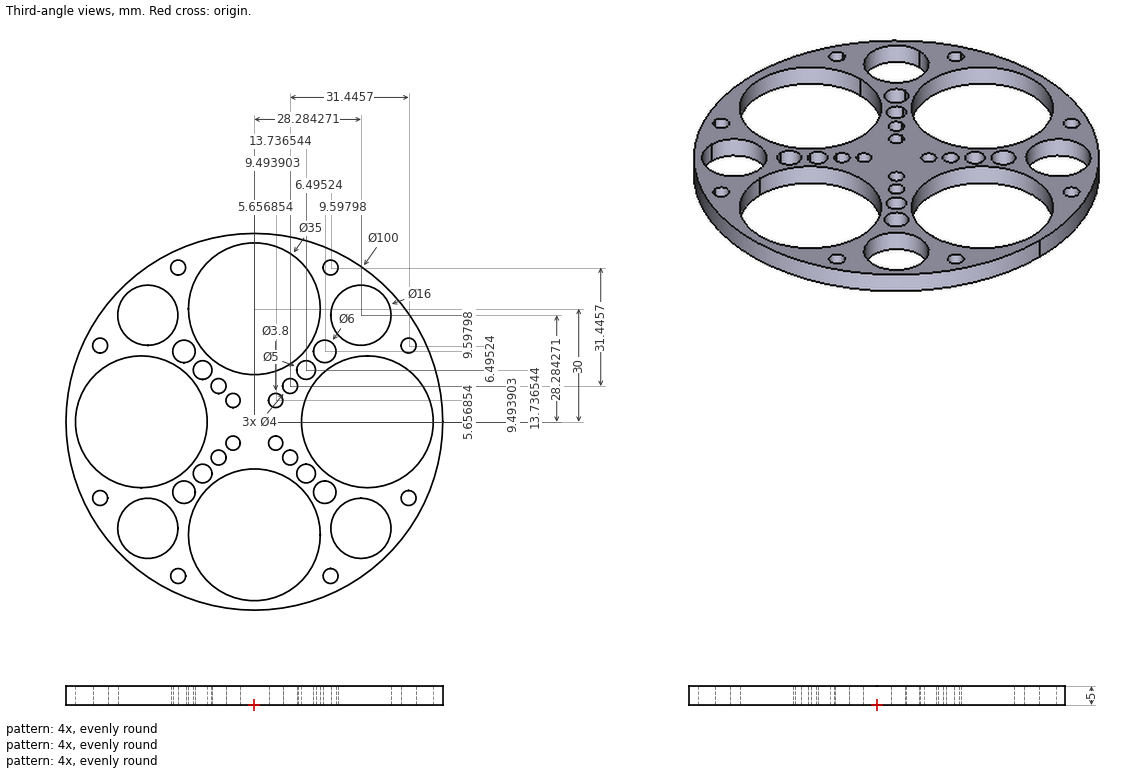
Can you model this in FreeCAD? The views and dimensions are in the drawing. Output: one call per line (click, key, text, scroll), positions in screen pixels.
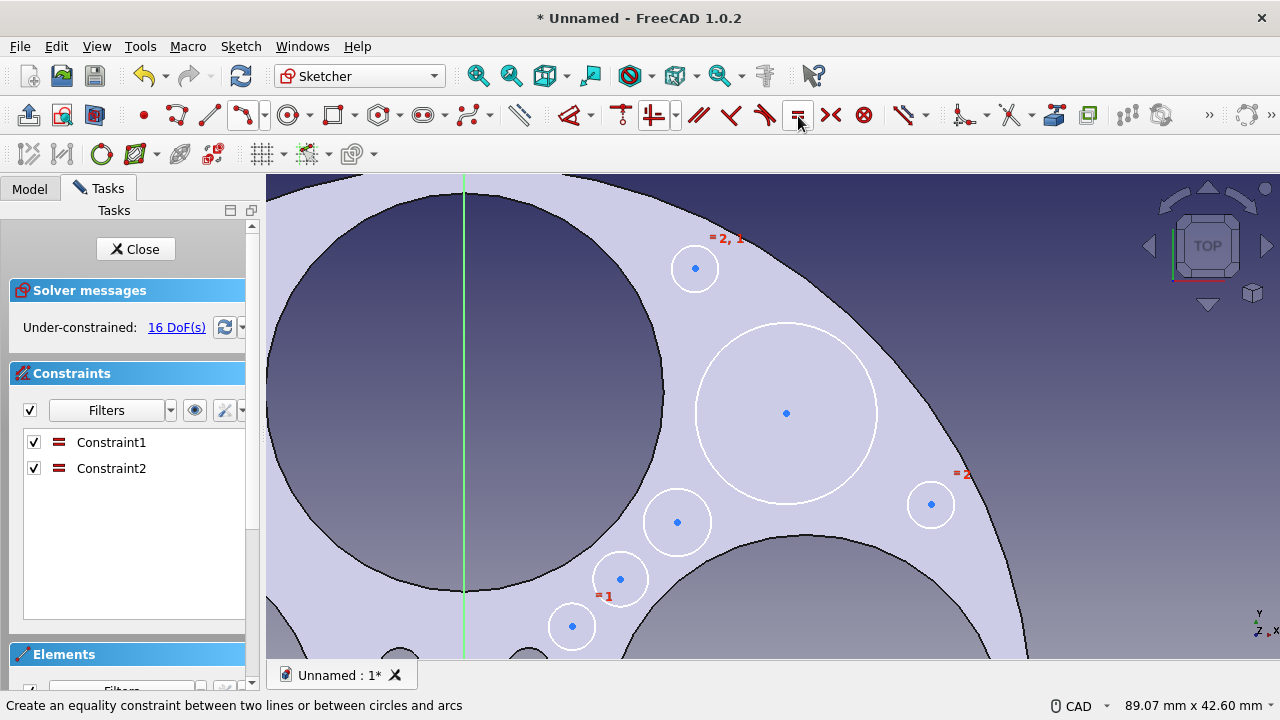
click(568, 116)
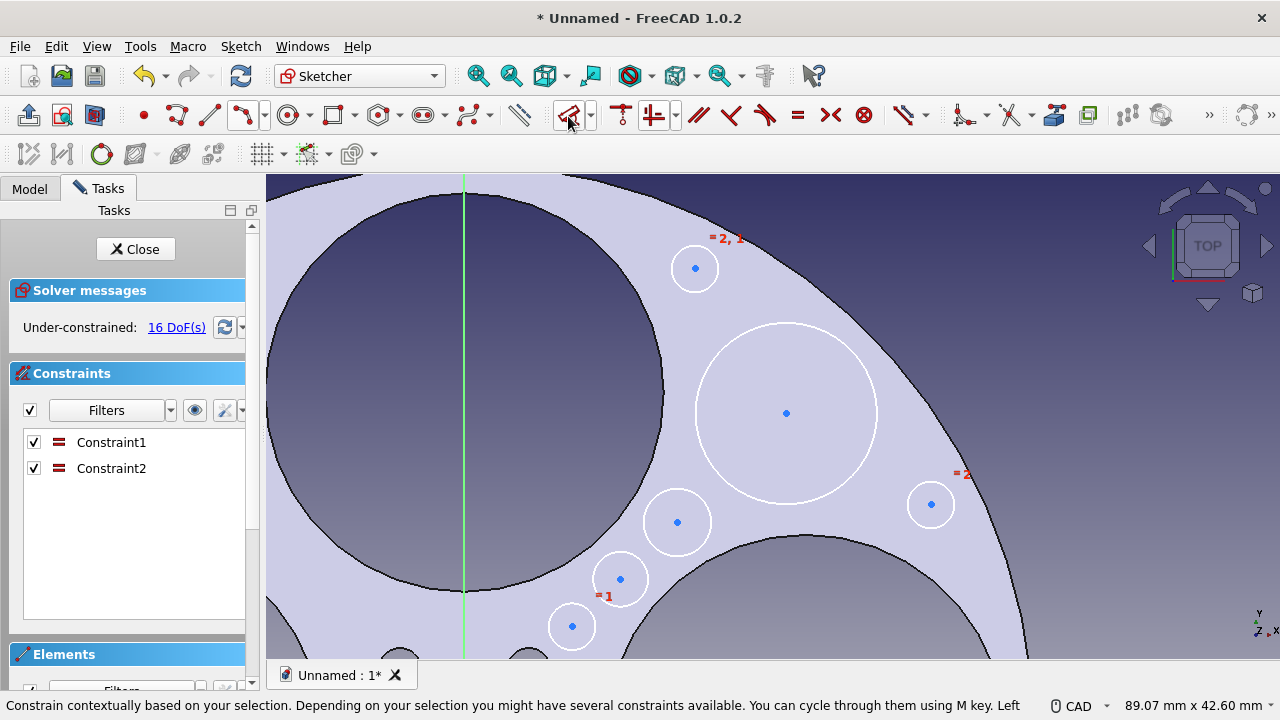
click(850, 349)
click(872, 326)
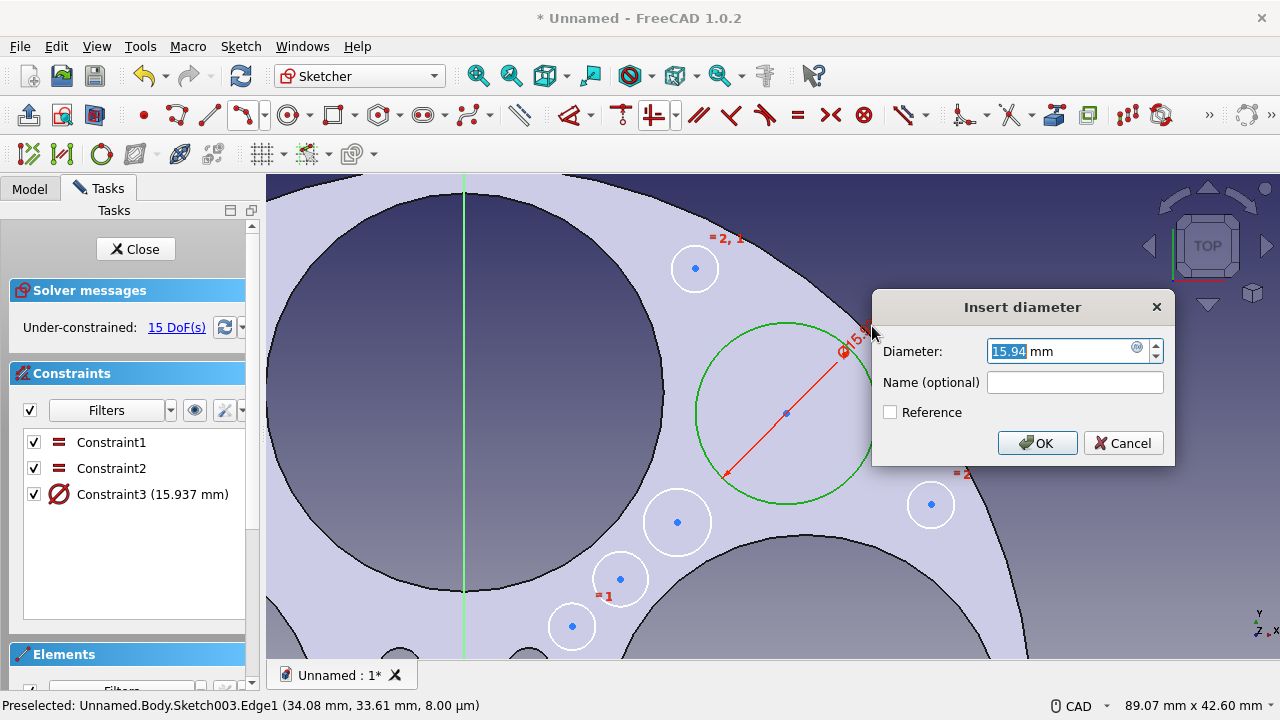
text(16)
key(Return)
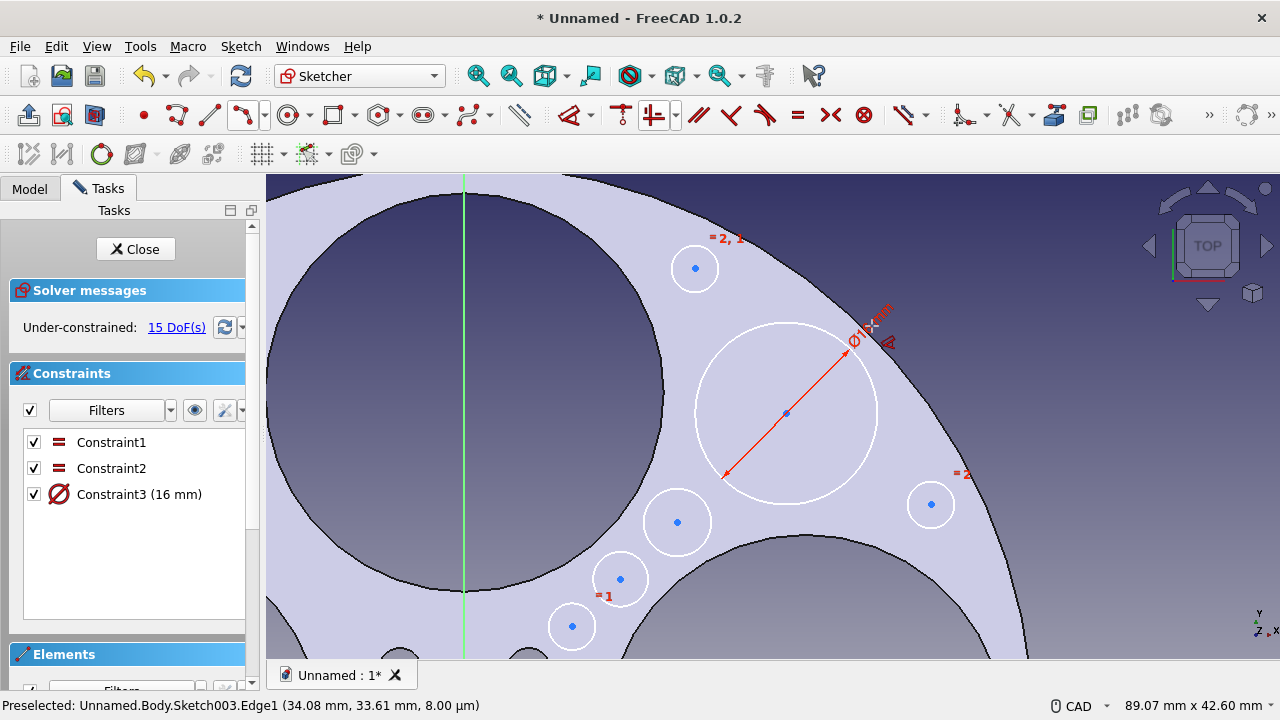
click(701, 499)
click(741, 537)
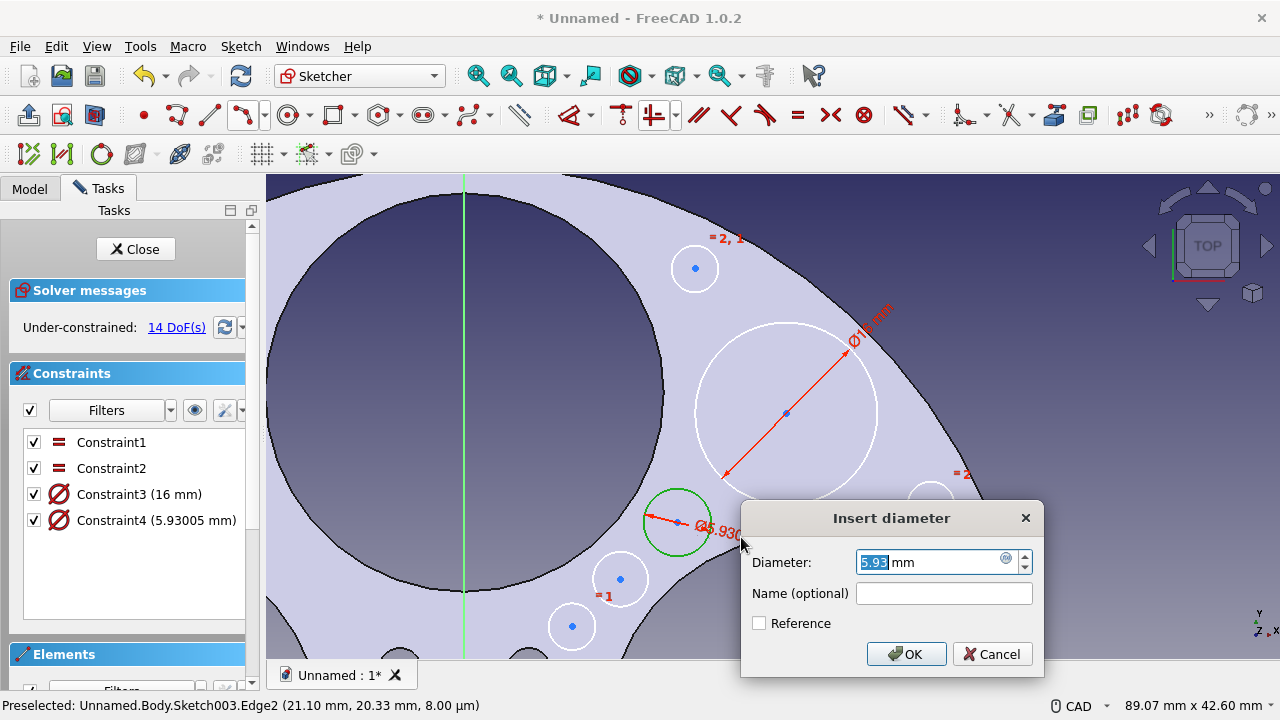
text(6)
key(Return)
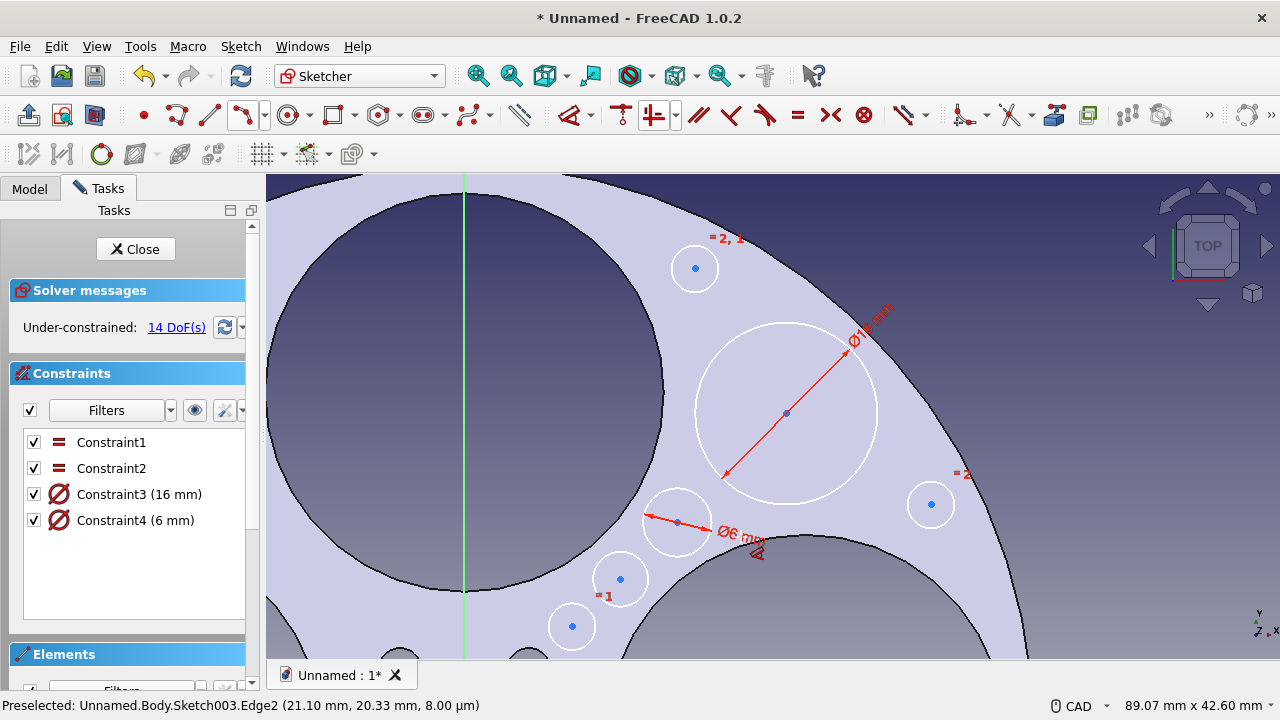
click(640, 560)
click(663, 537)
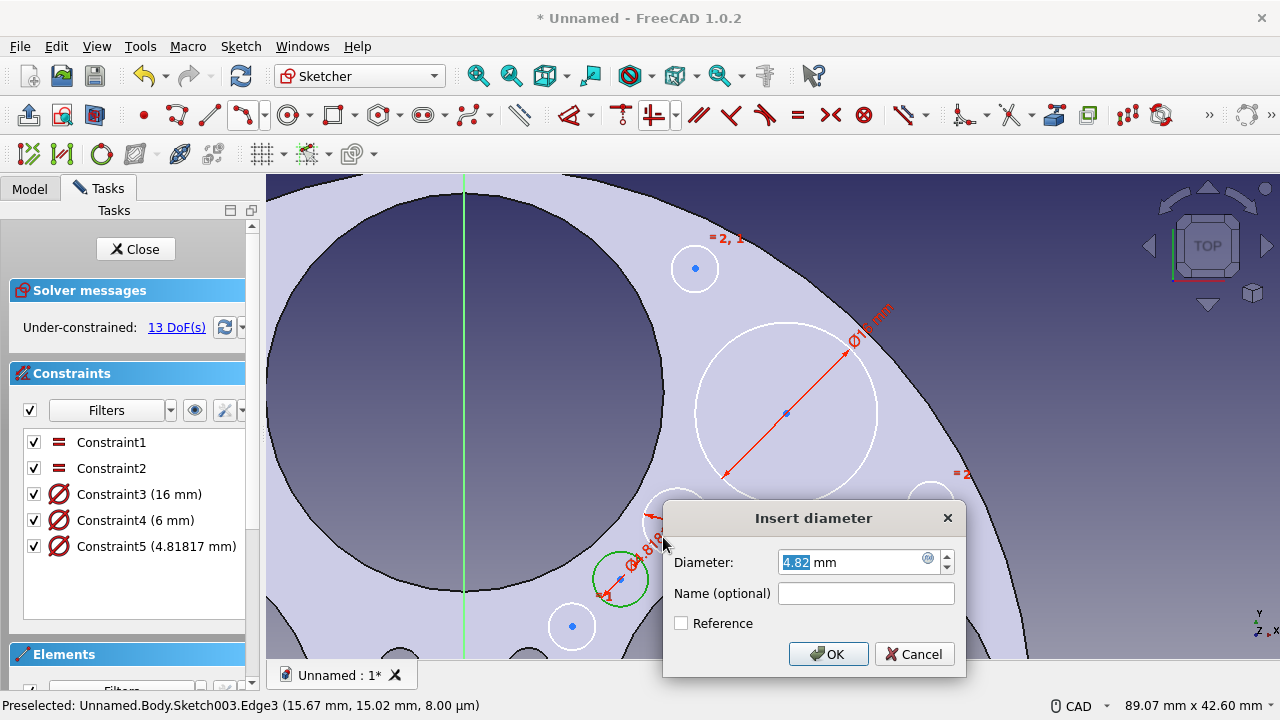
text(5)
key(Return)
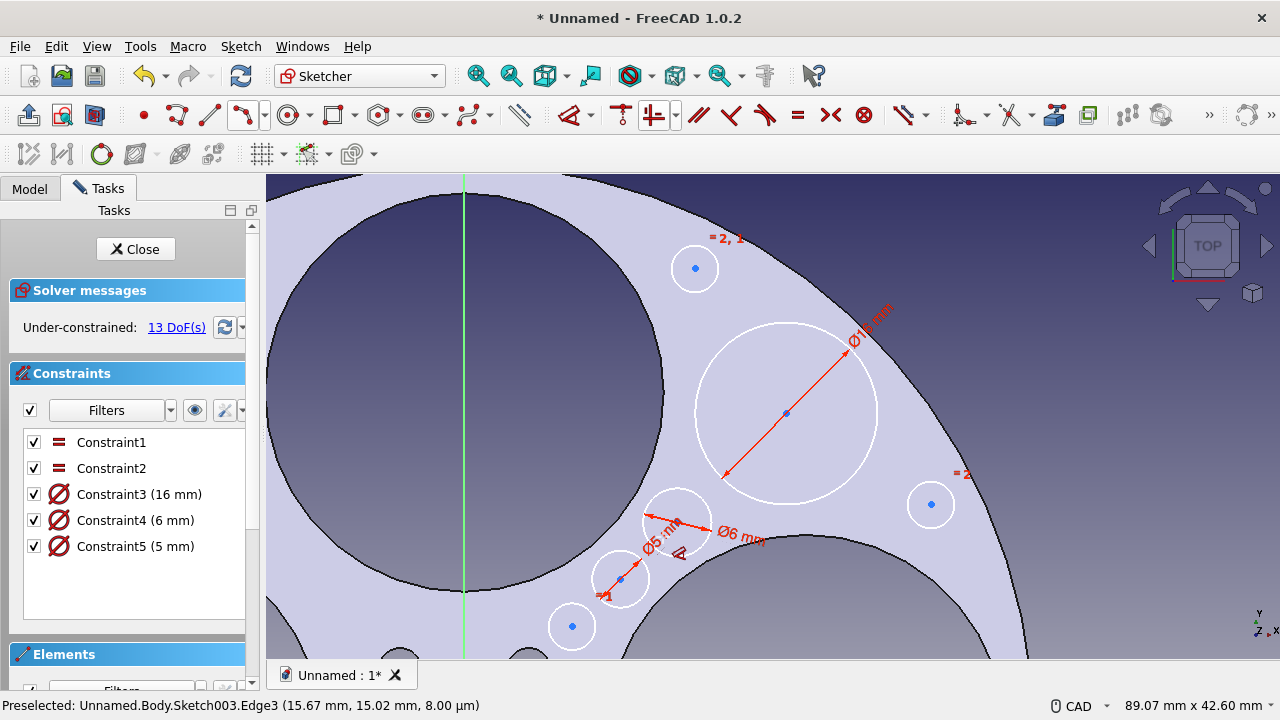
click(589, 610)
click(612, 587)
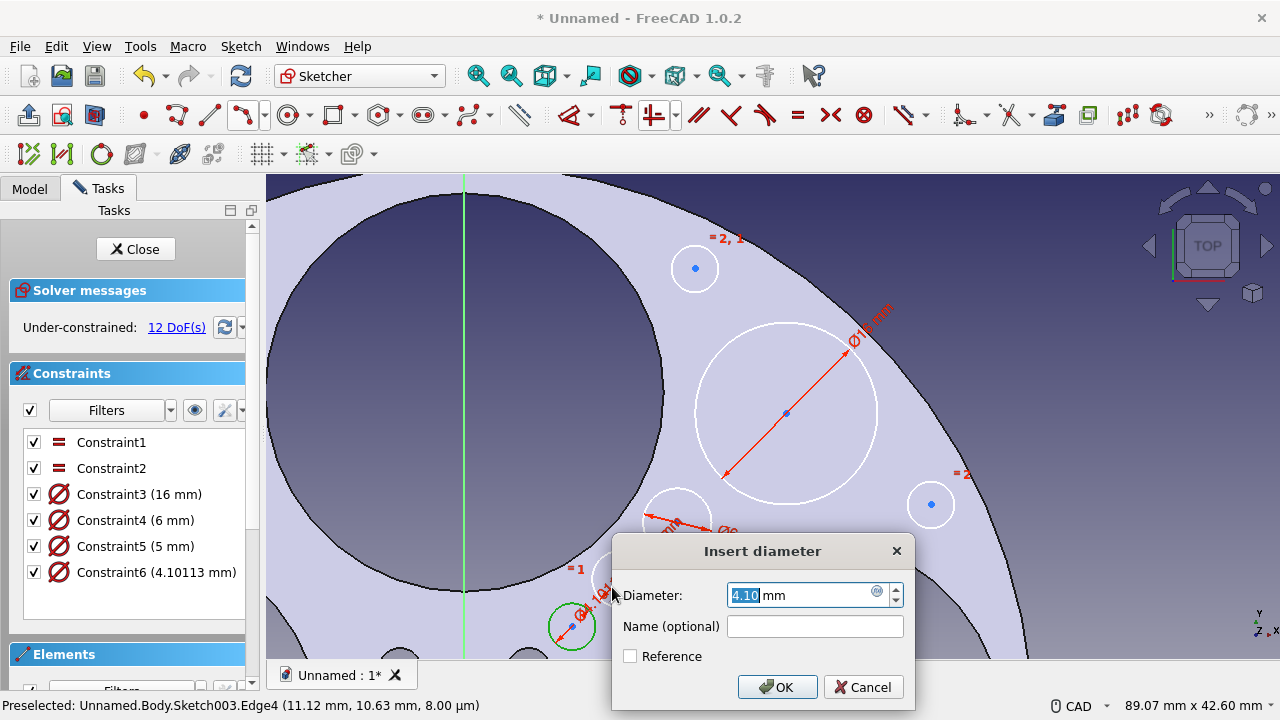
text(4)
key(Return)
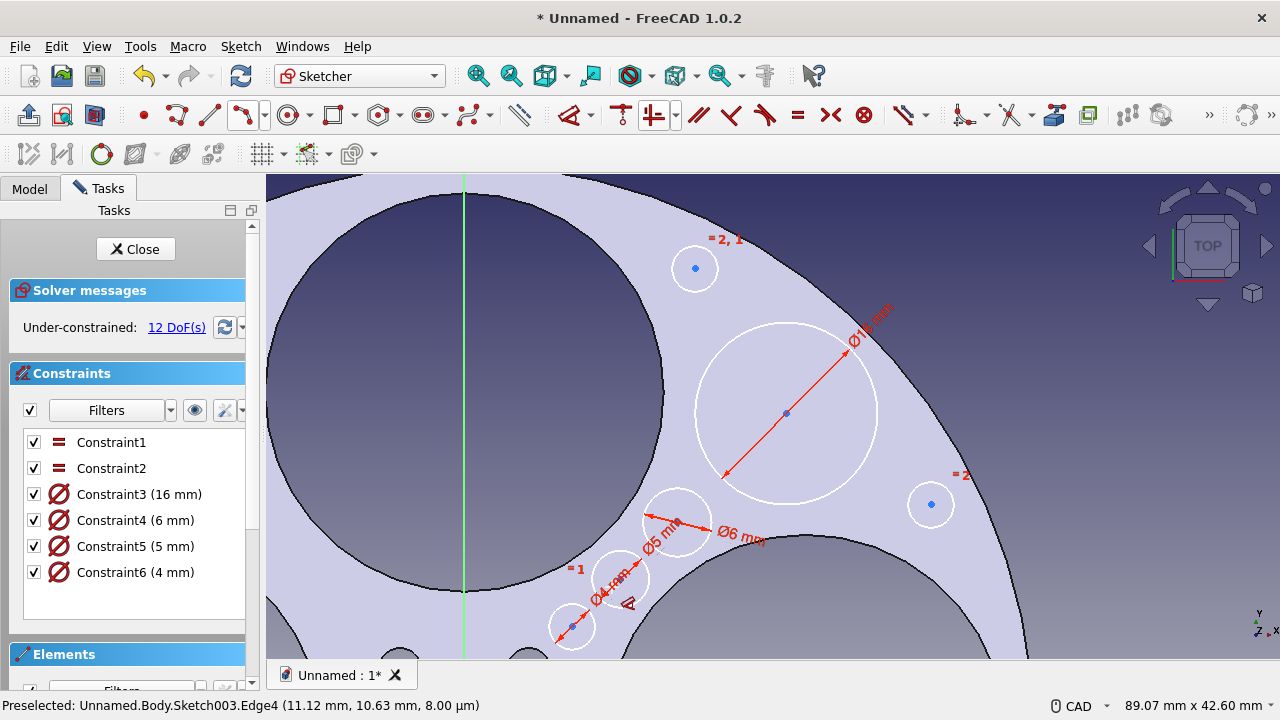
click(572, 627)
click(518, 593)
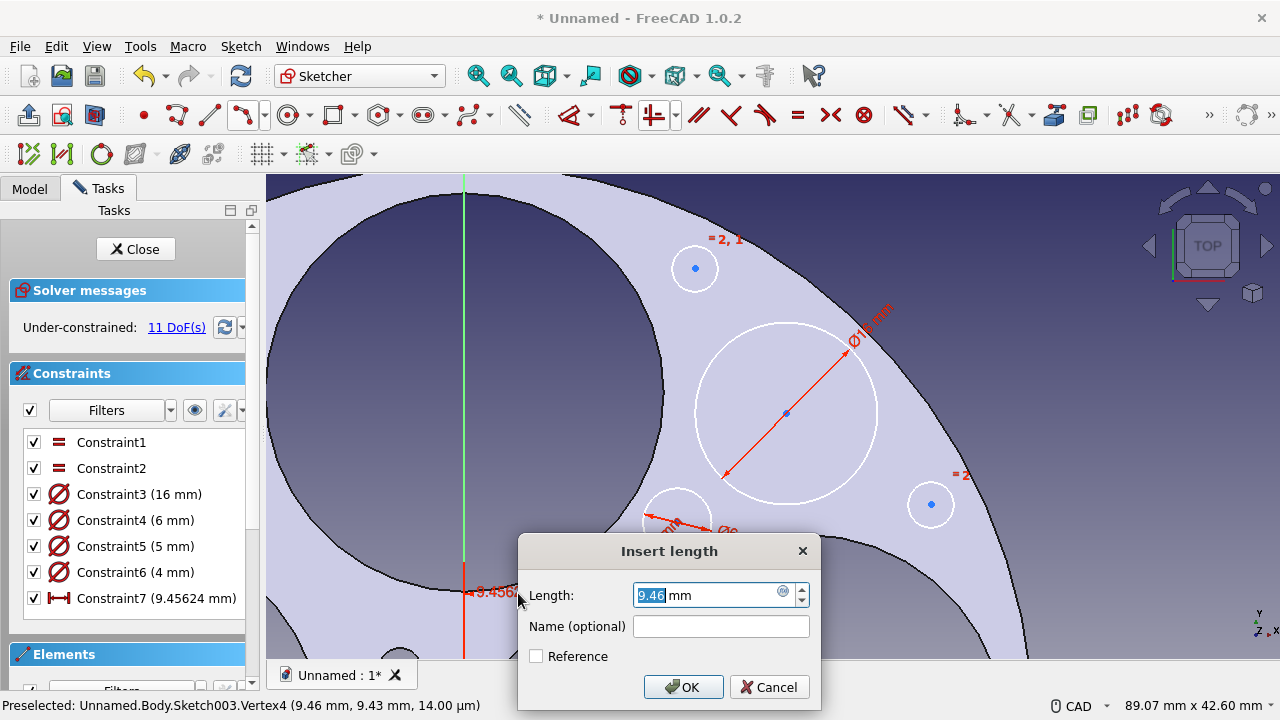
text(9.493903)
key(Return)